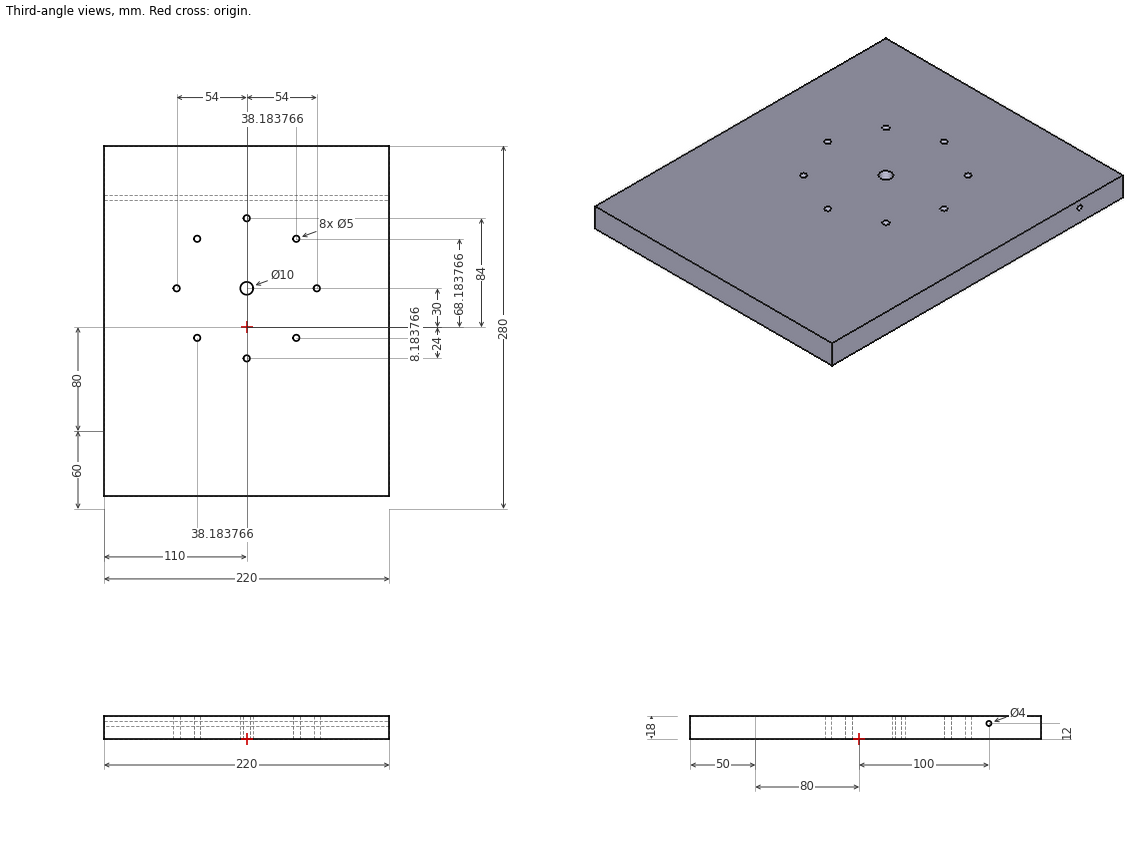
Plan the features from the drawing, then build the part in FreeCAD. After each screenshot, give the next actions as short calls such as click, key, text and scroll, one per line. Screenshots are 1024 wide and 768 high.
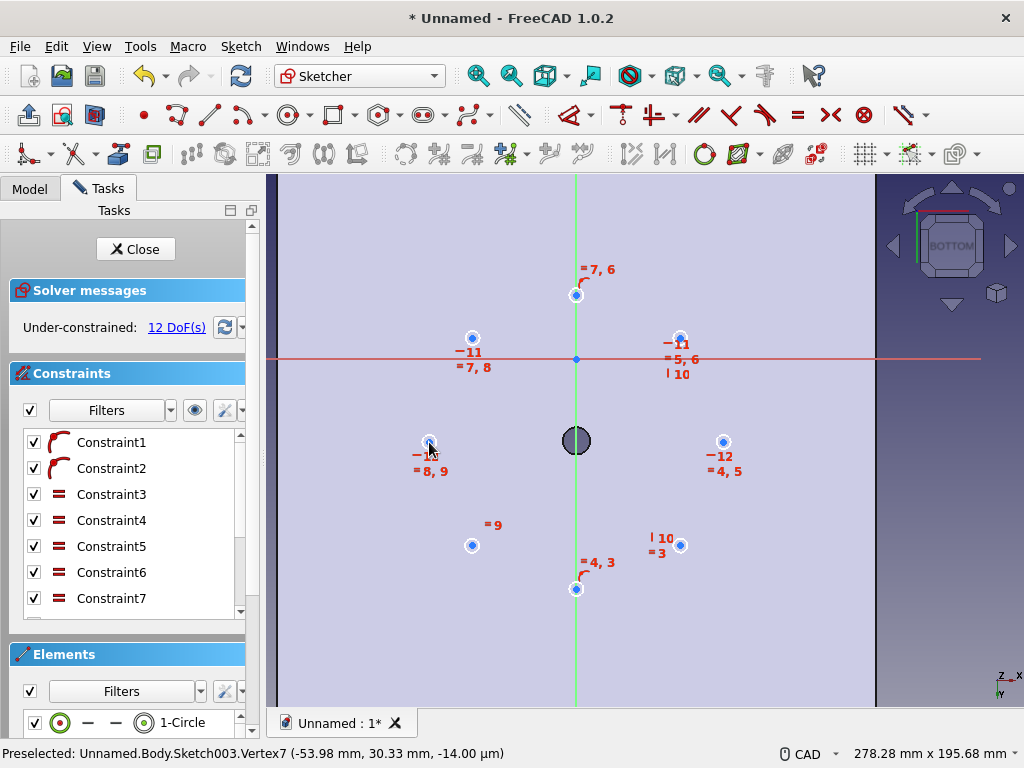
click(473, 338)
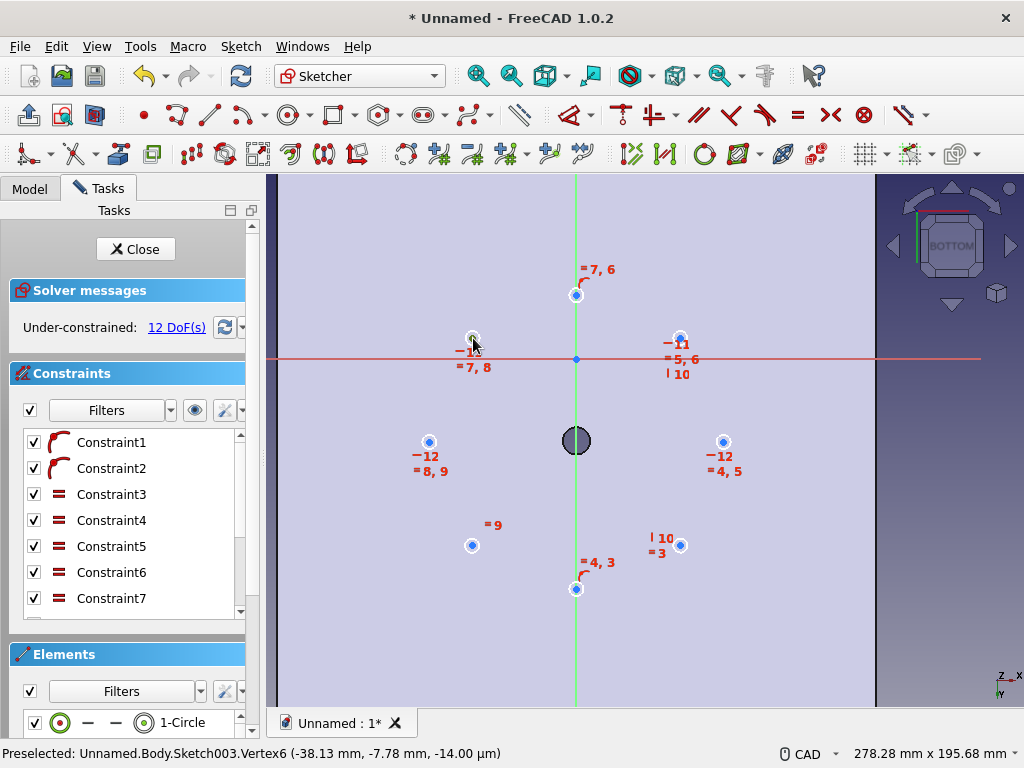
click(472, 546)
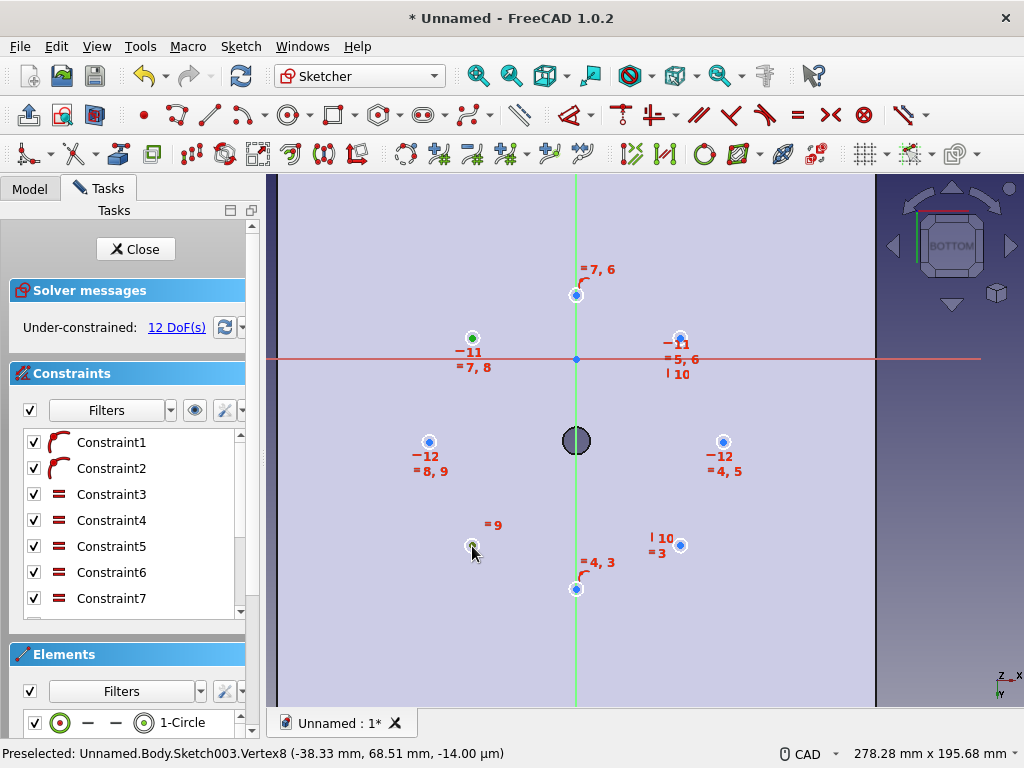
key(v)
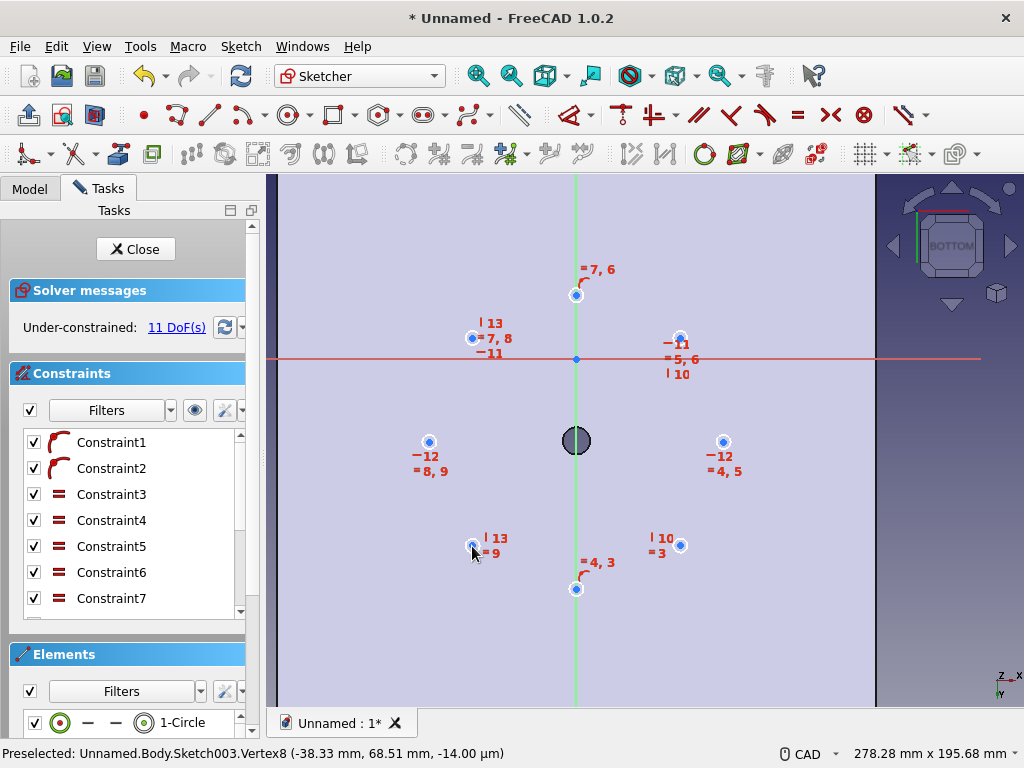
click(680, 546)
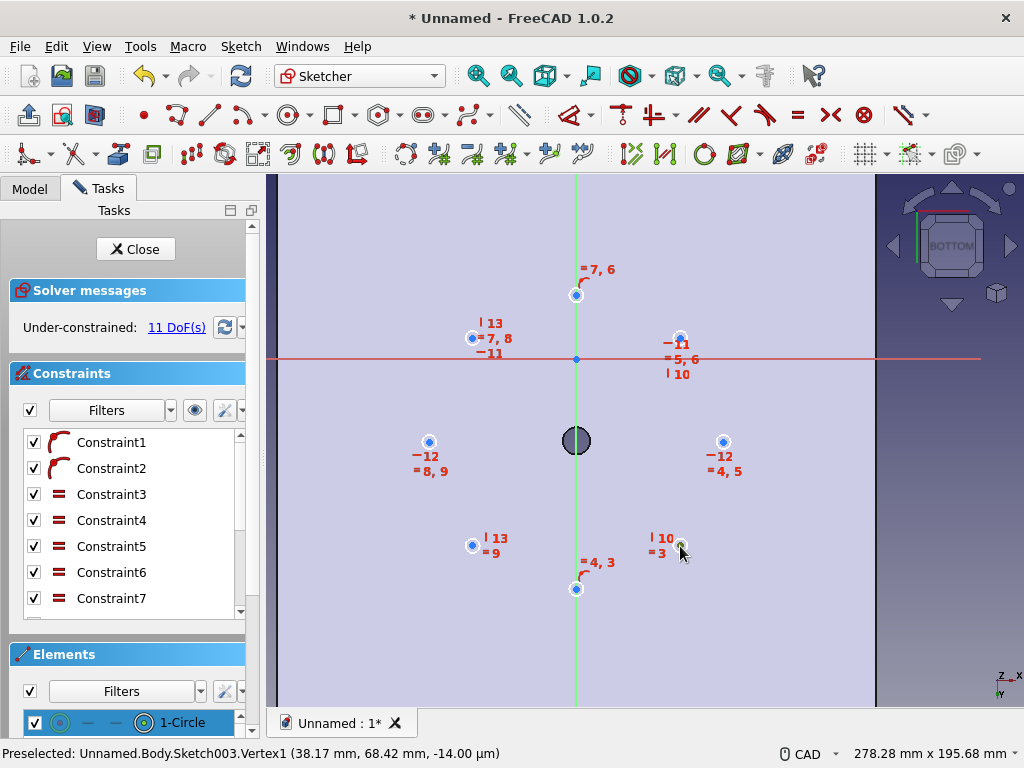
click(473, 546)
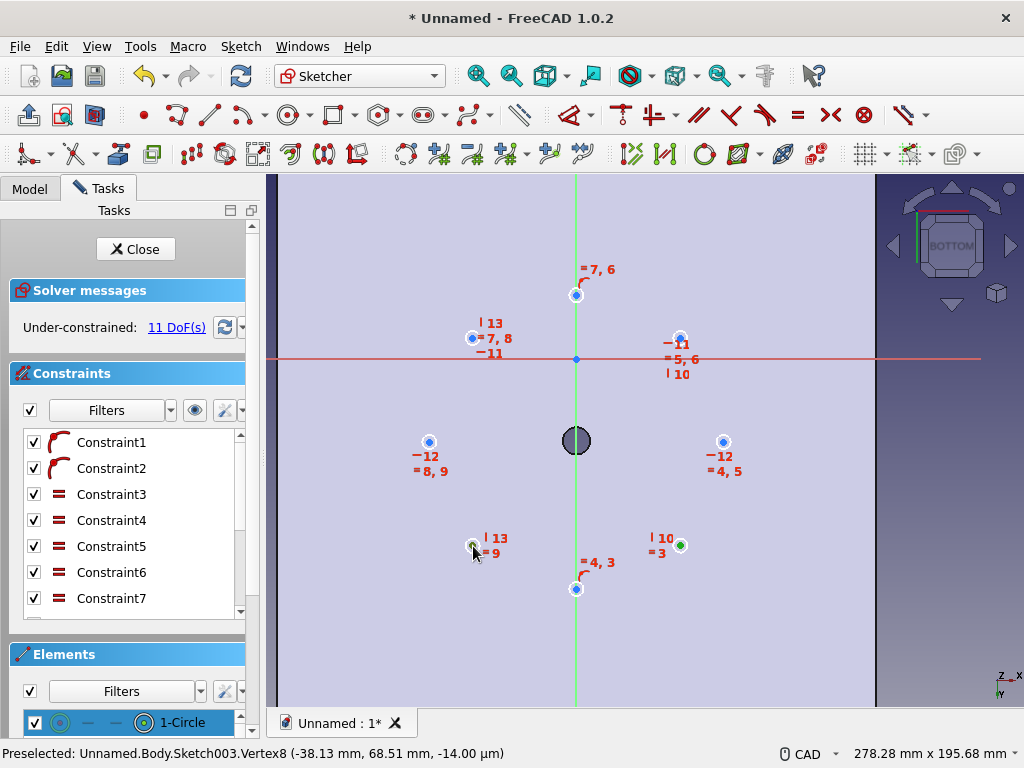
key(h)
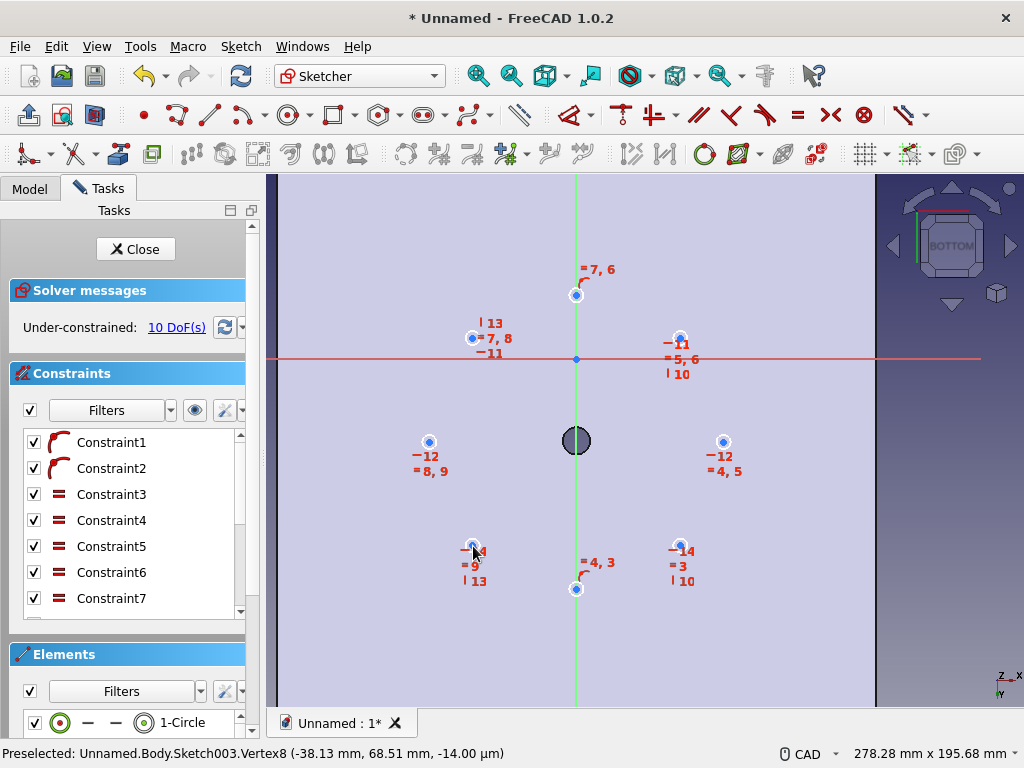
key(d)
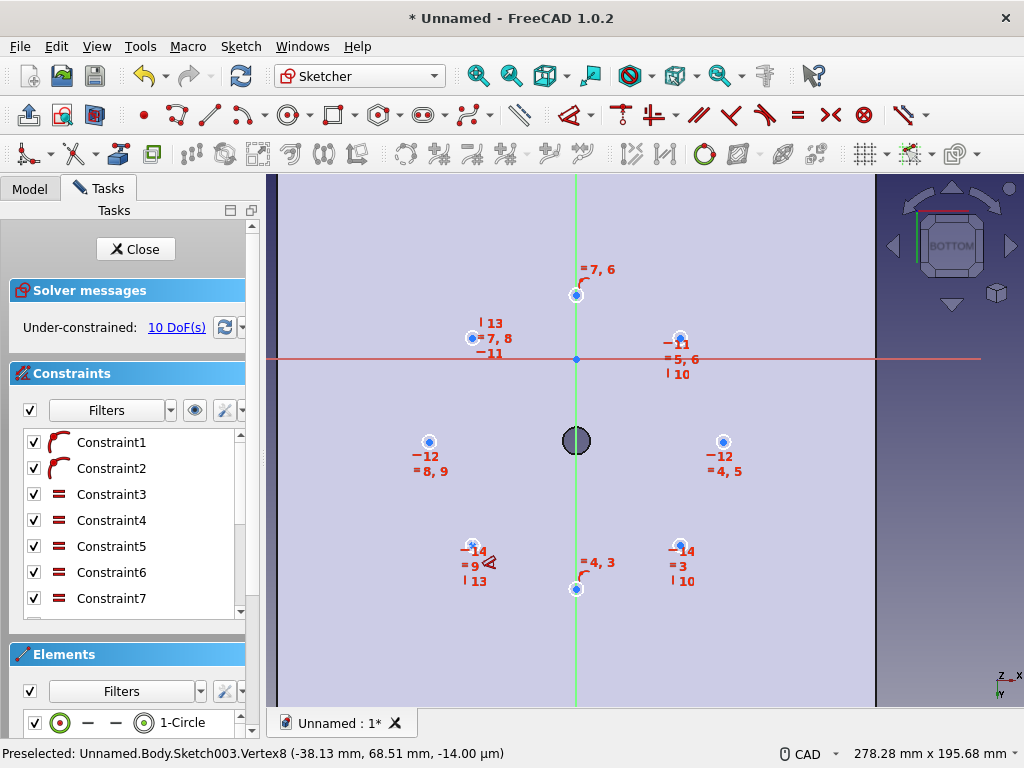
scroll(680, 553, up, 6)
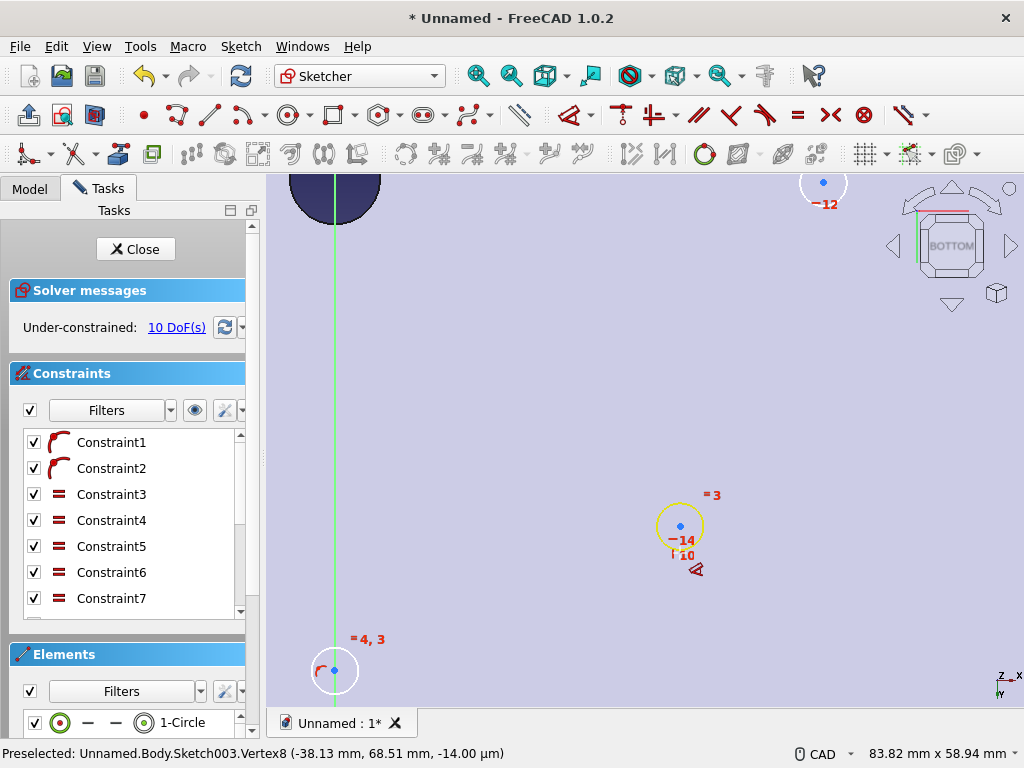
click(680, 550)
click(680, 582)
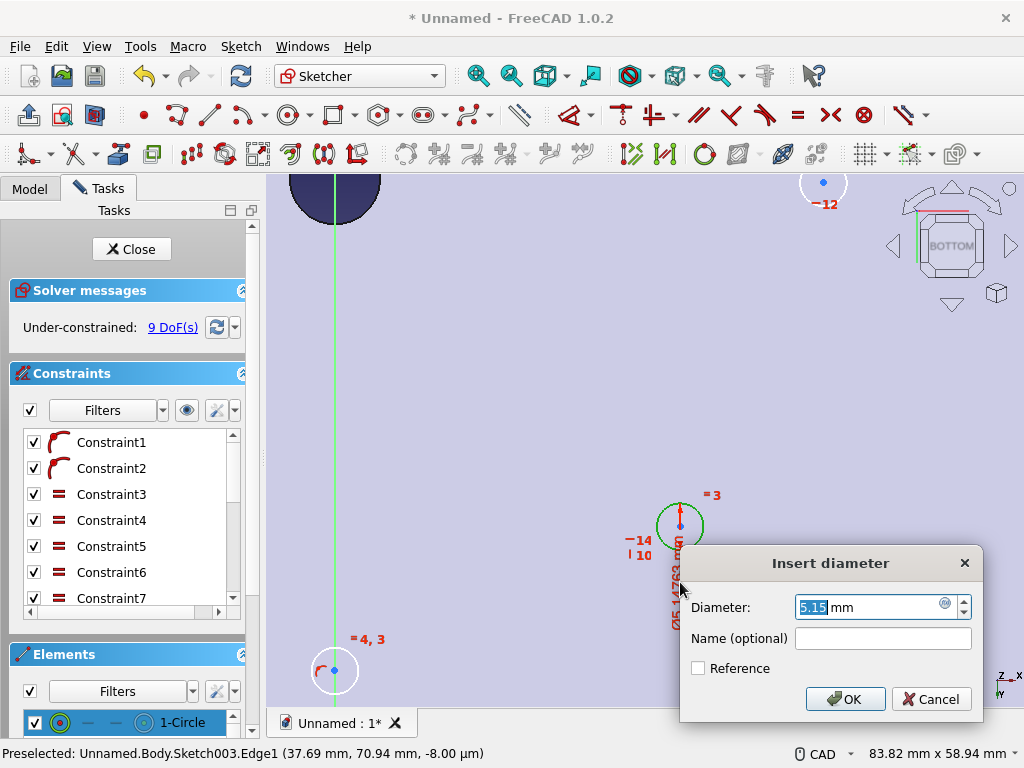
text(5)
key(Return)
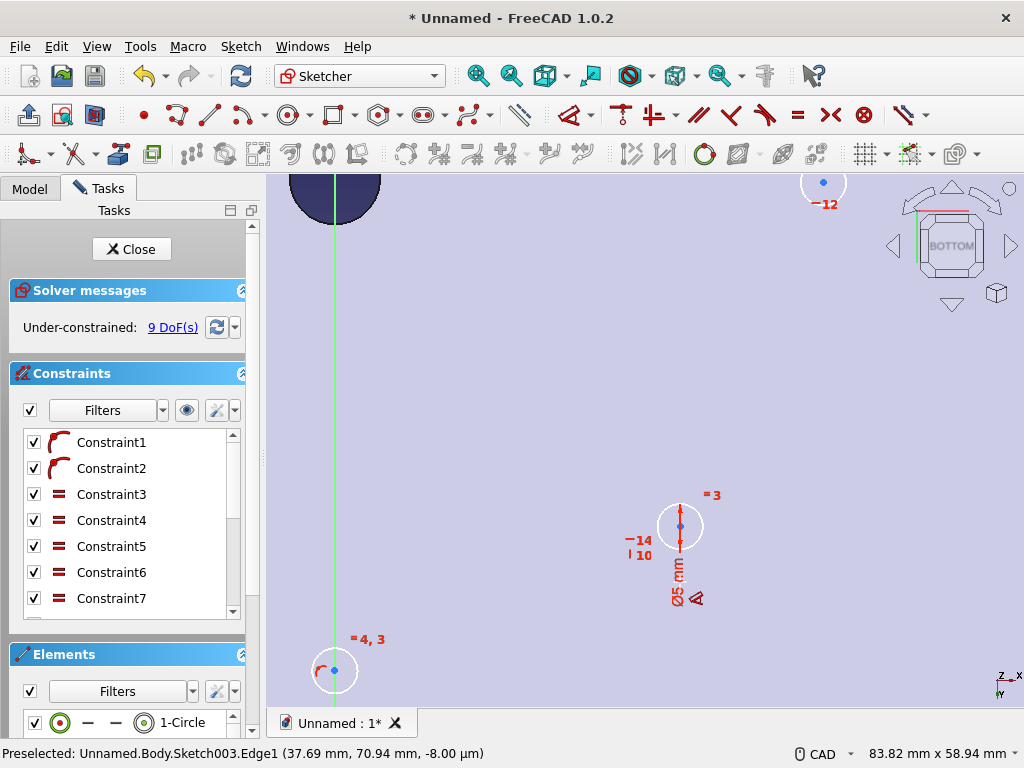
click(335, 671)
click(369, 436)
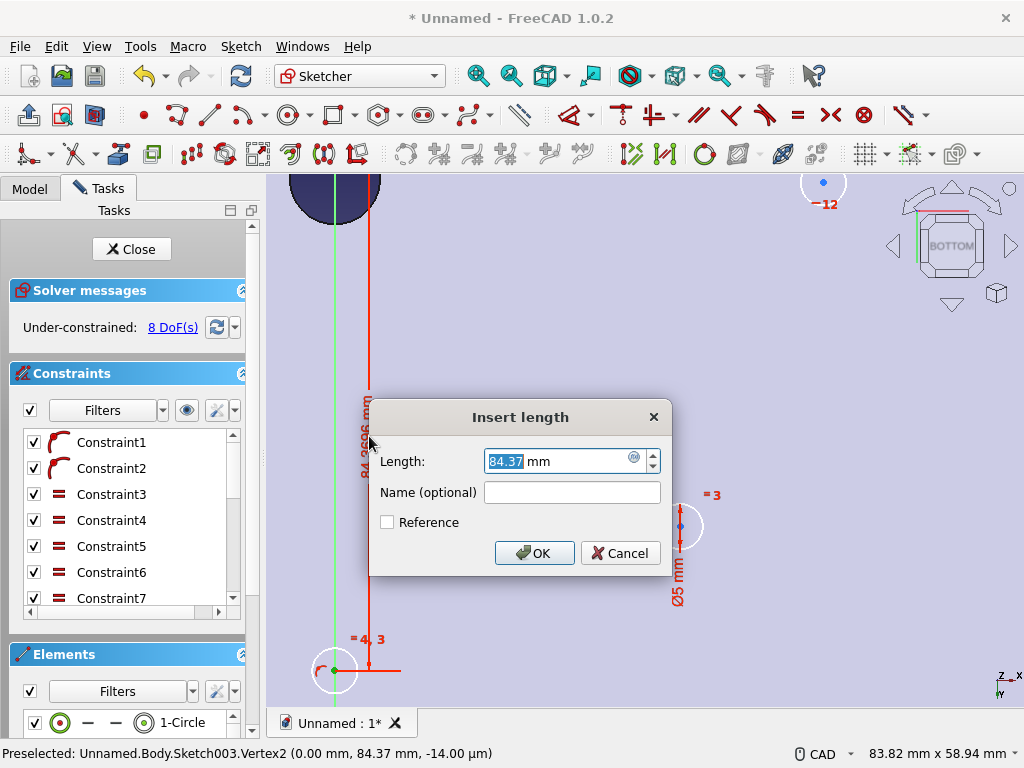
text(84)
key(Return)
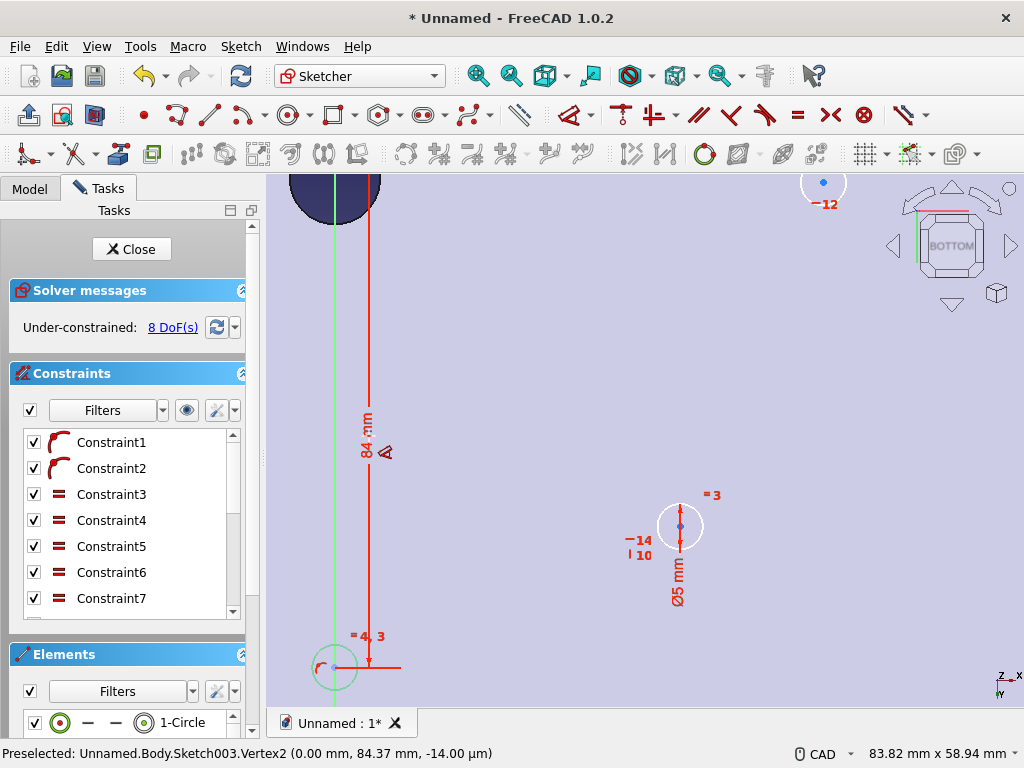
scroll(681, 553, down, 6)